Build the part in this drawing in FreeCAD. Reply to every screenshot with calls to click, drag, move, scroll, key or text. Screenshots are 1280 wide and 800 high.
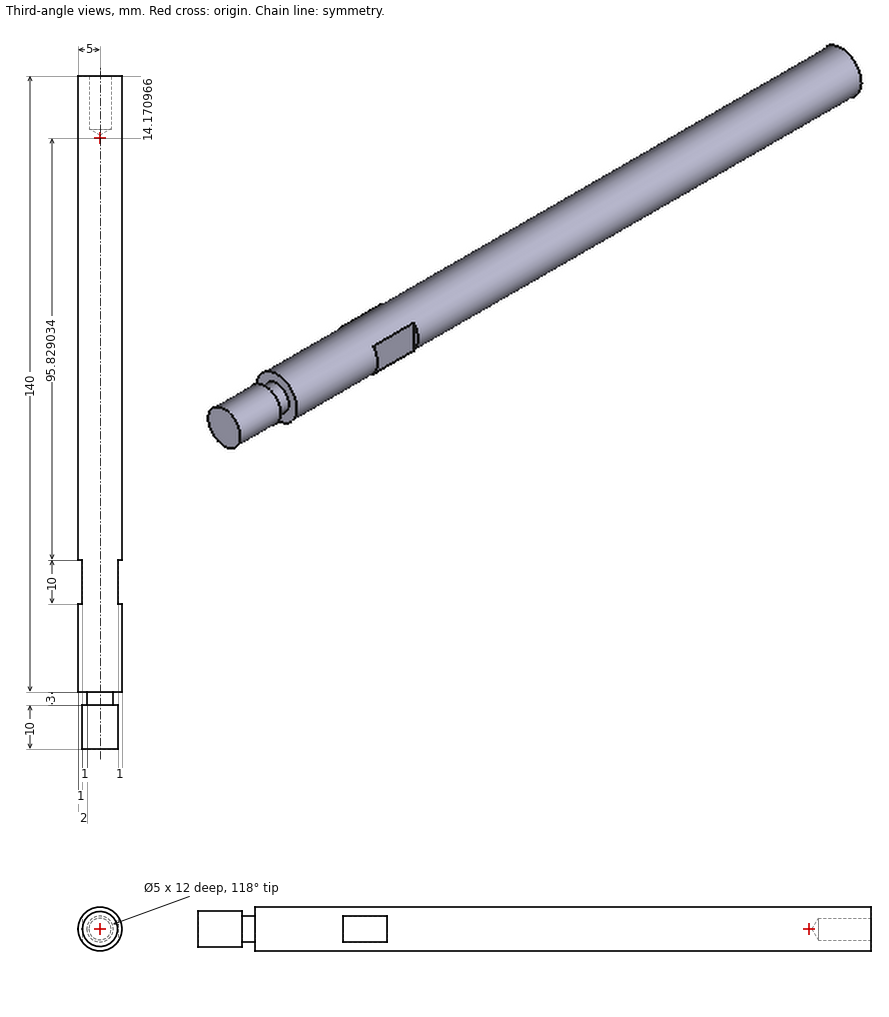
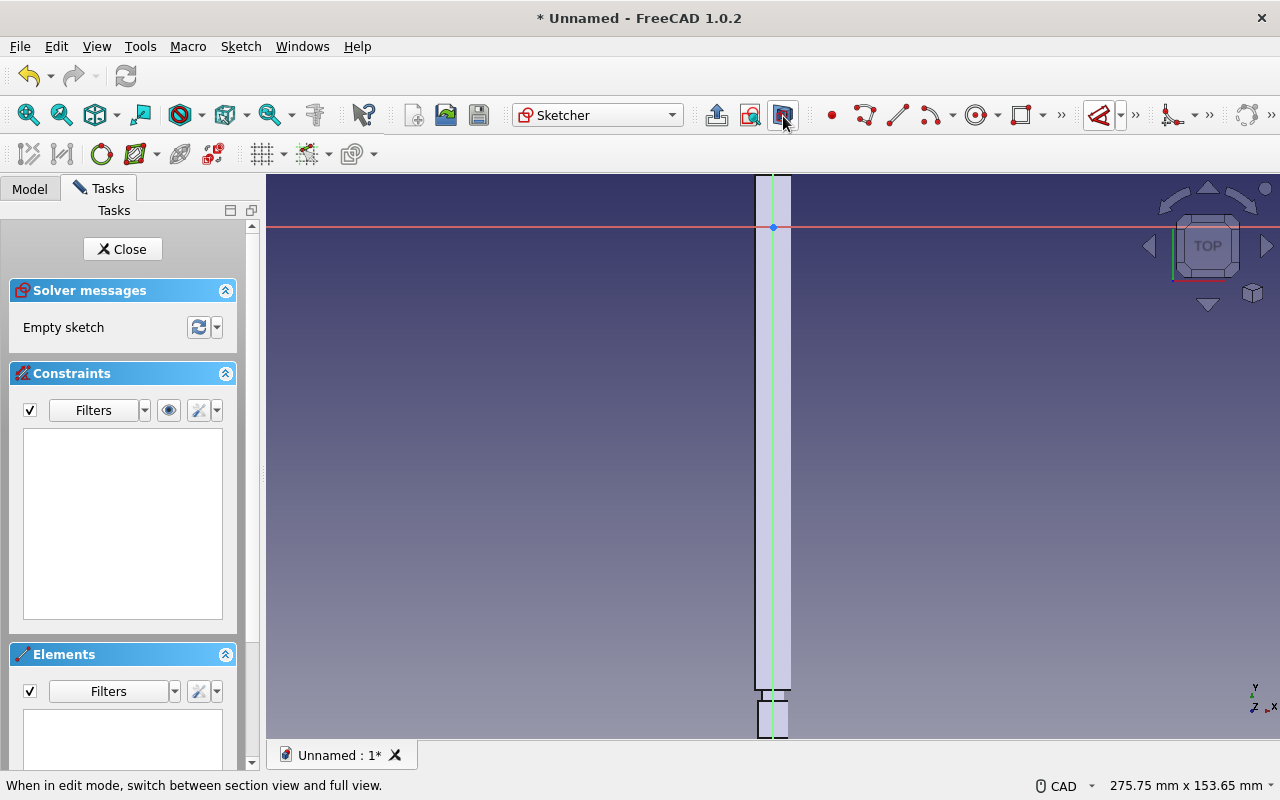
scroll(782, 616, up, 11)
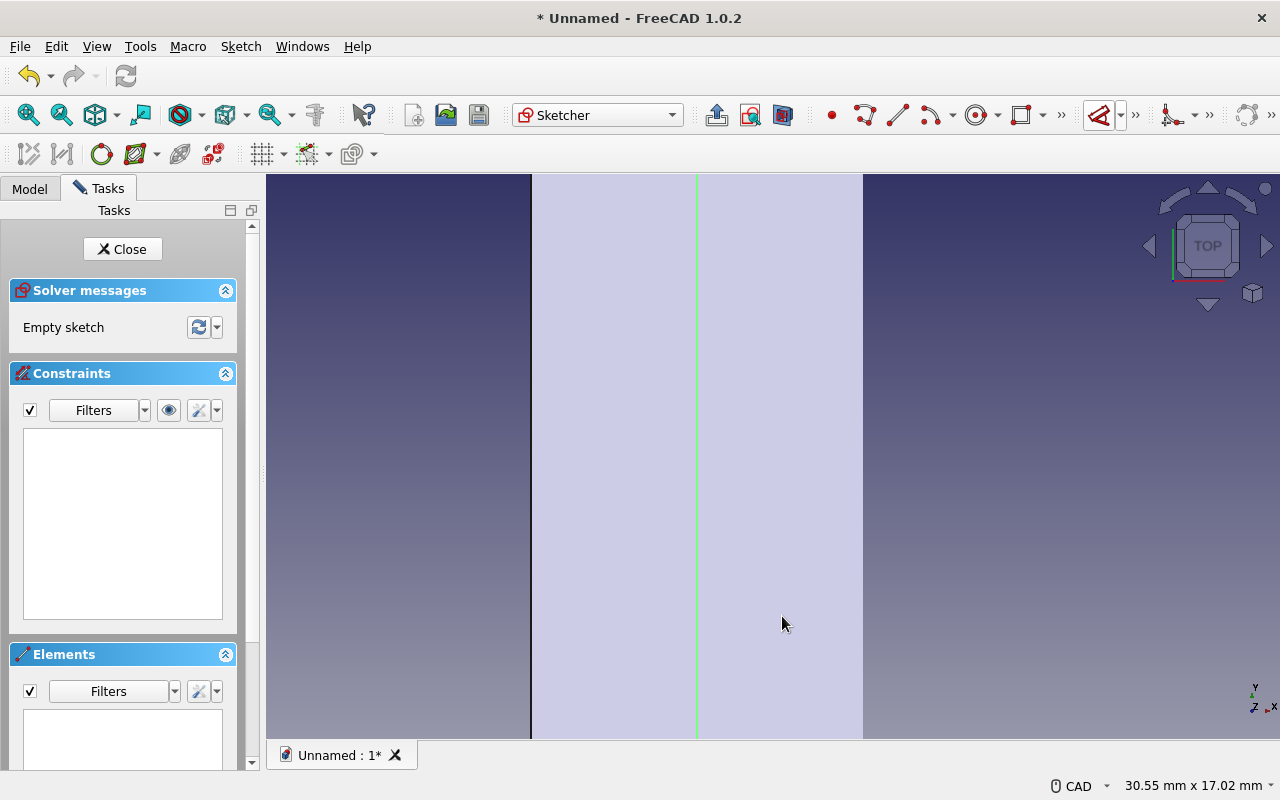
click(1020, 116)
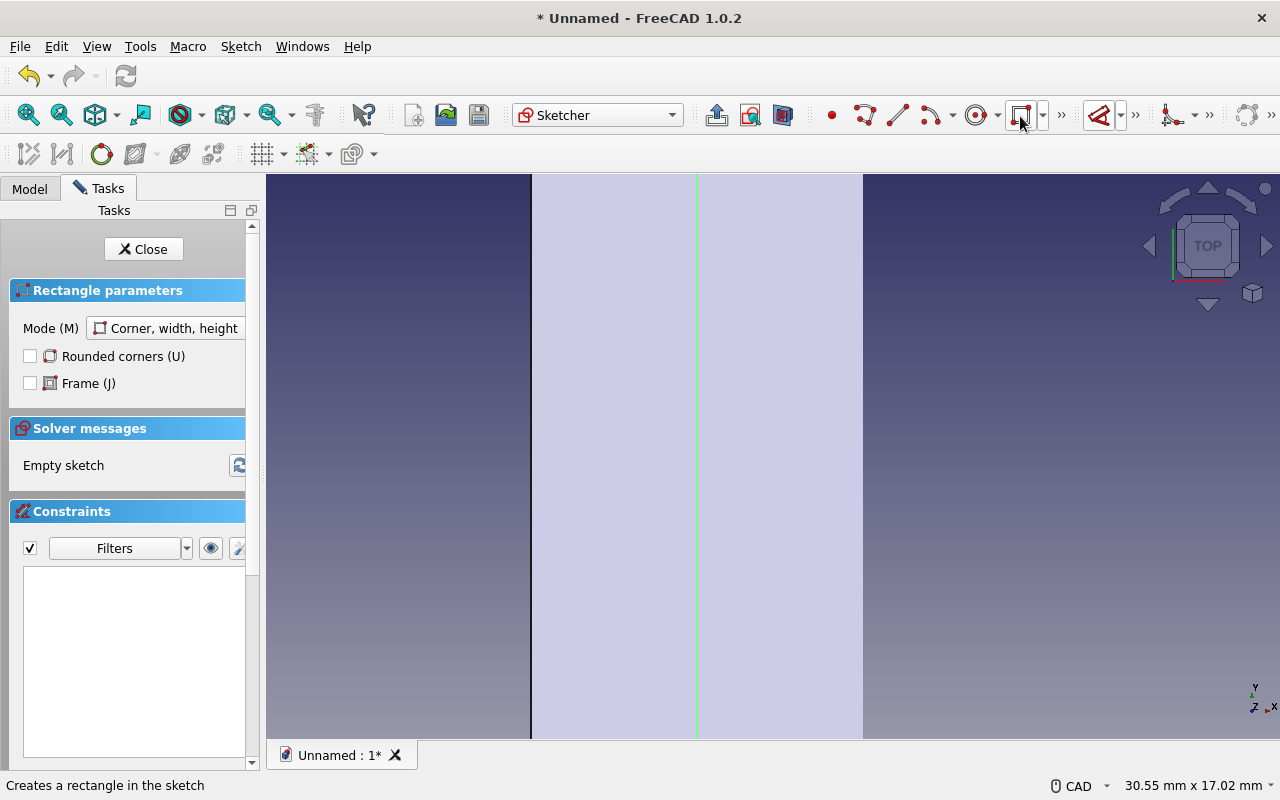
click(531, 282)
move(564, 614)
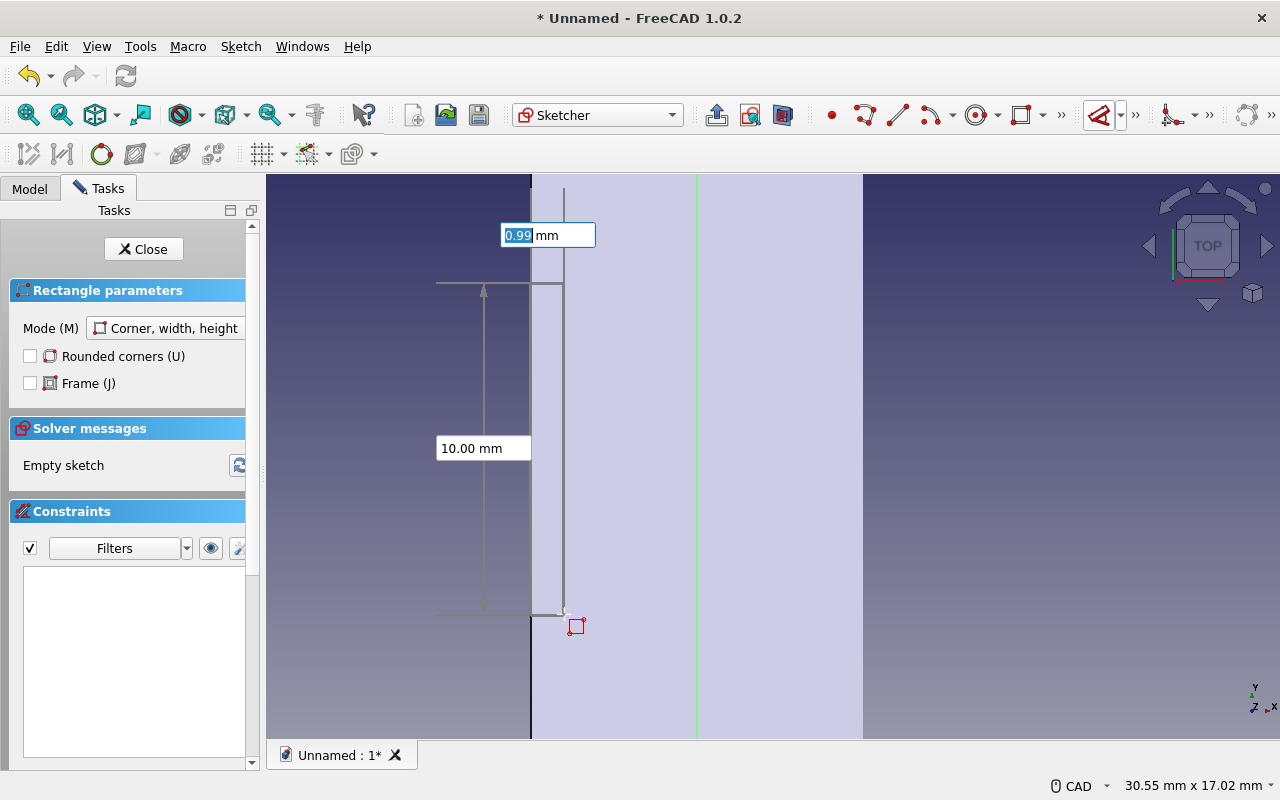
text(1)
key(Tab)
text(10)
key(Return)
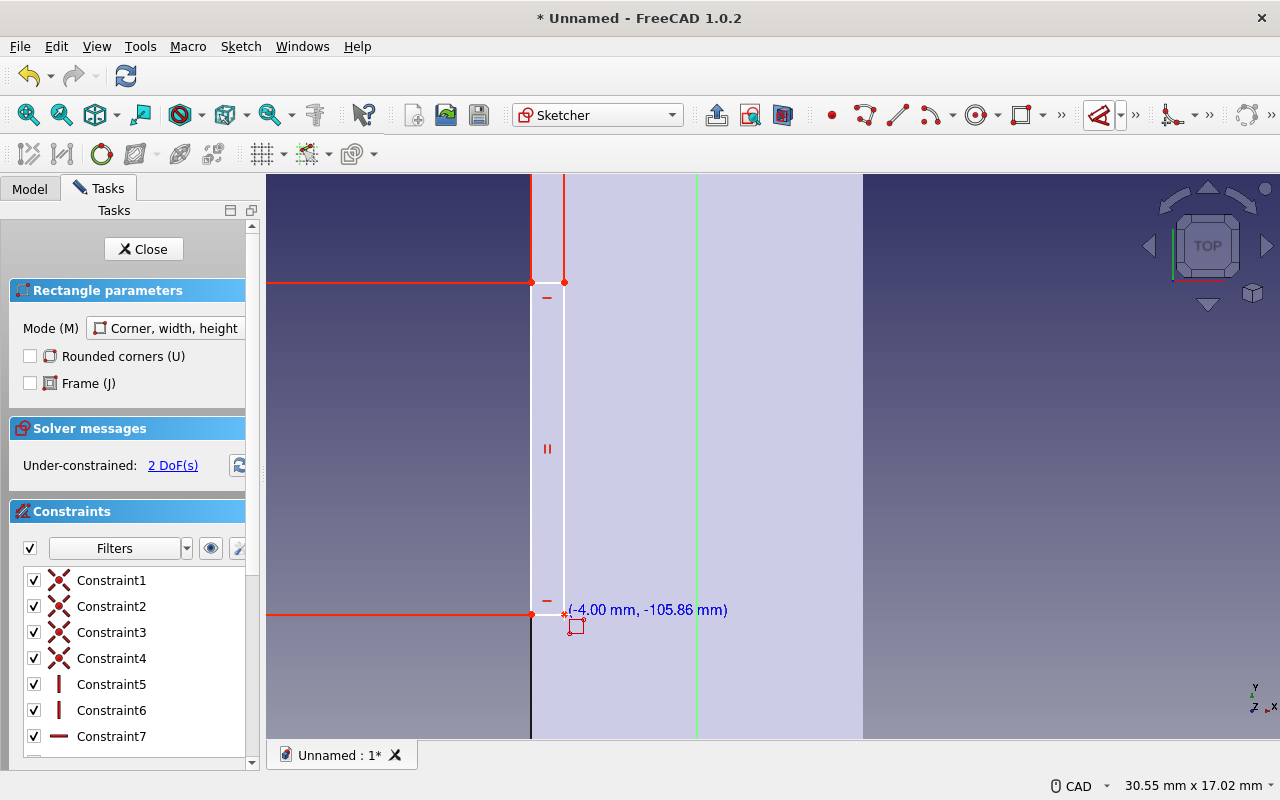
click(829, 282)
move(863, 614)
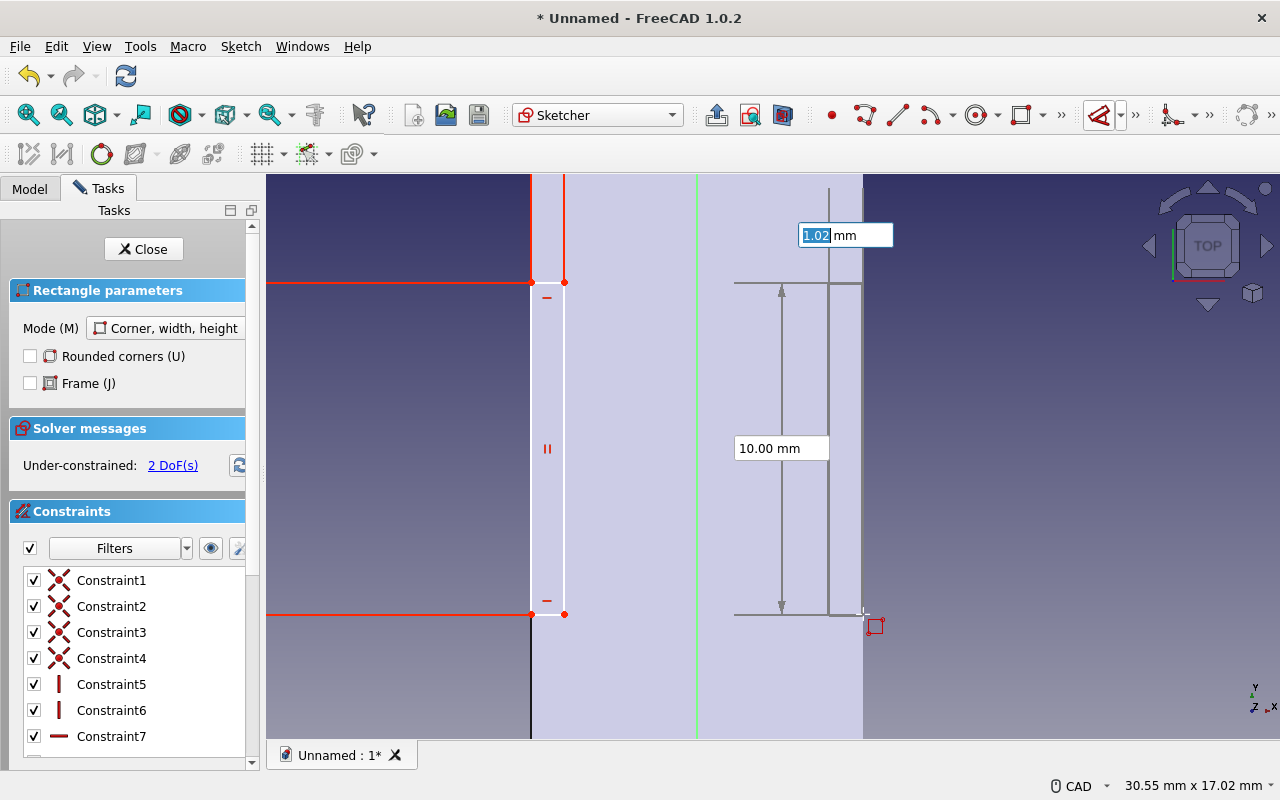
text(1)
key(Tab)
text(10)
key(Return)
key(Escape)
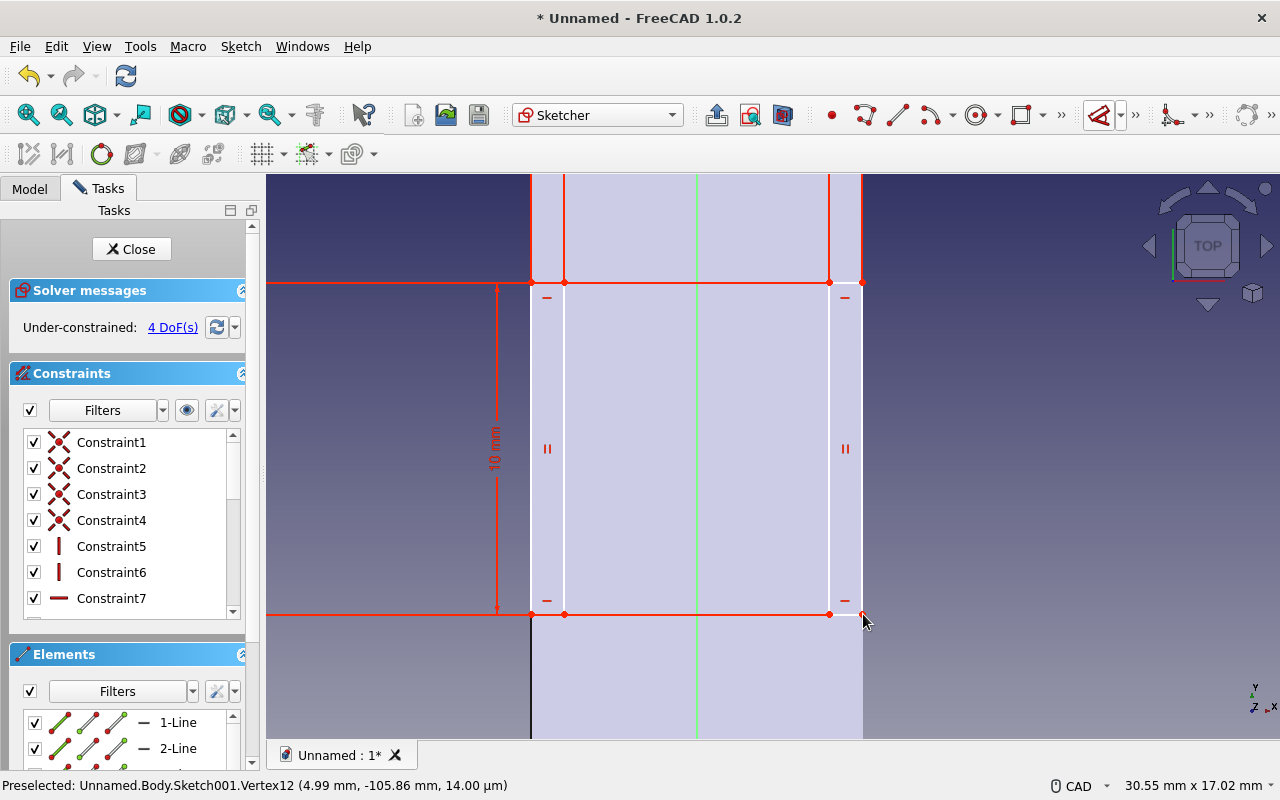
click(564, 283)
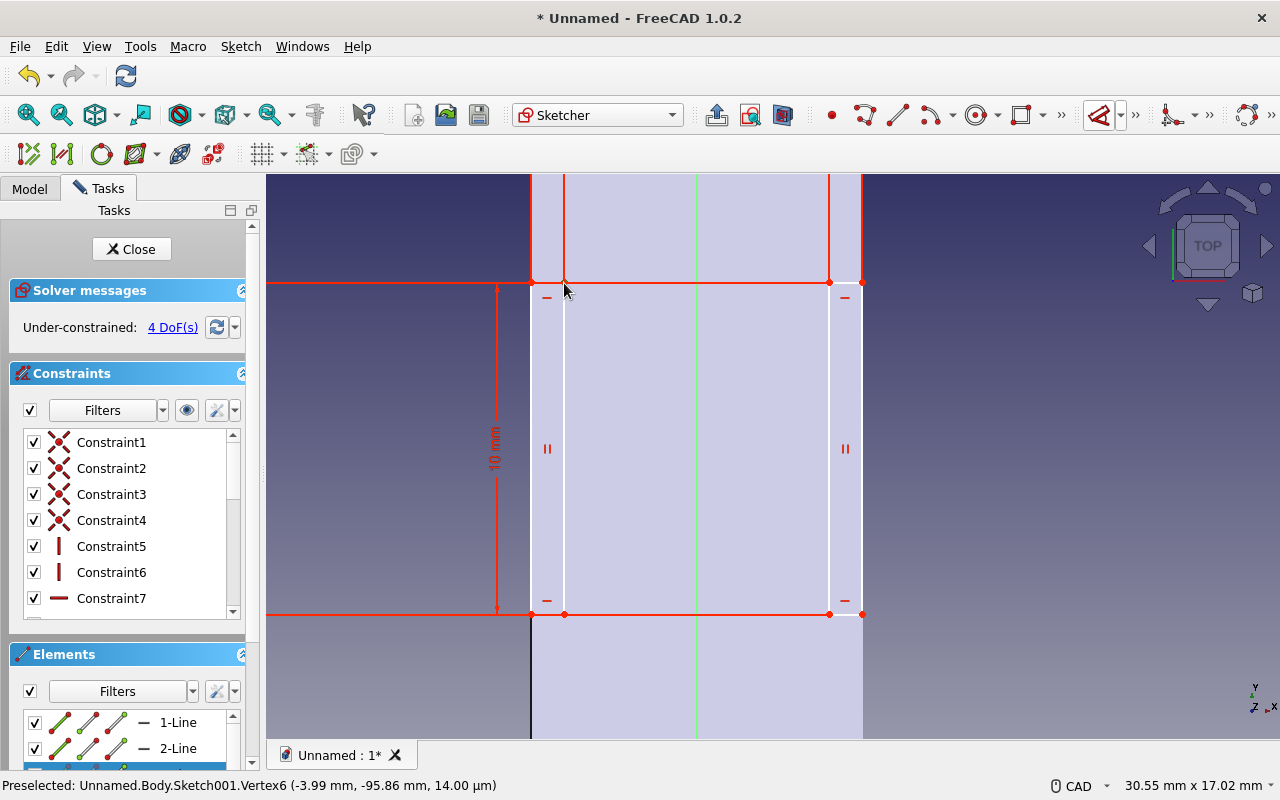
click(829, 283)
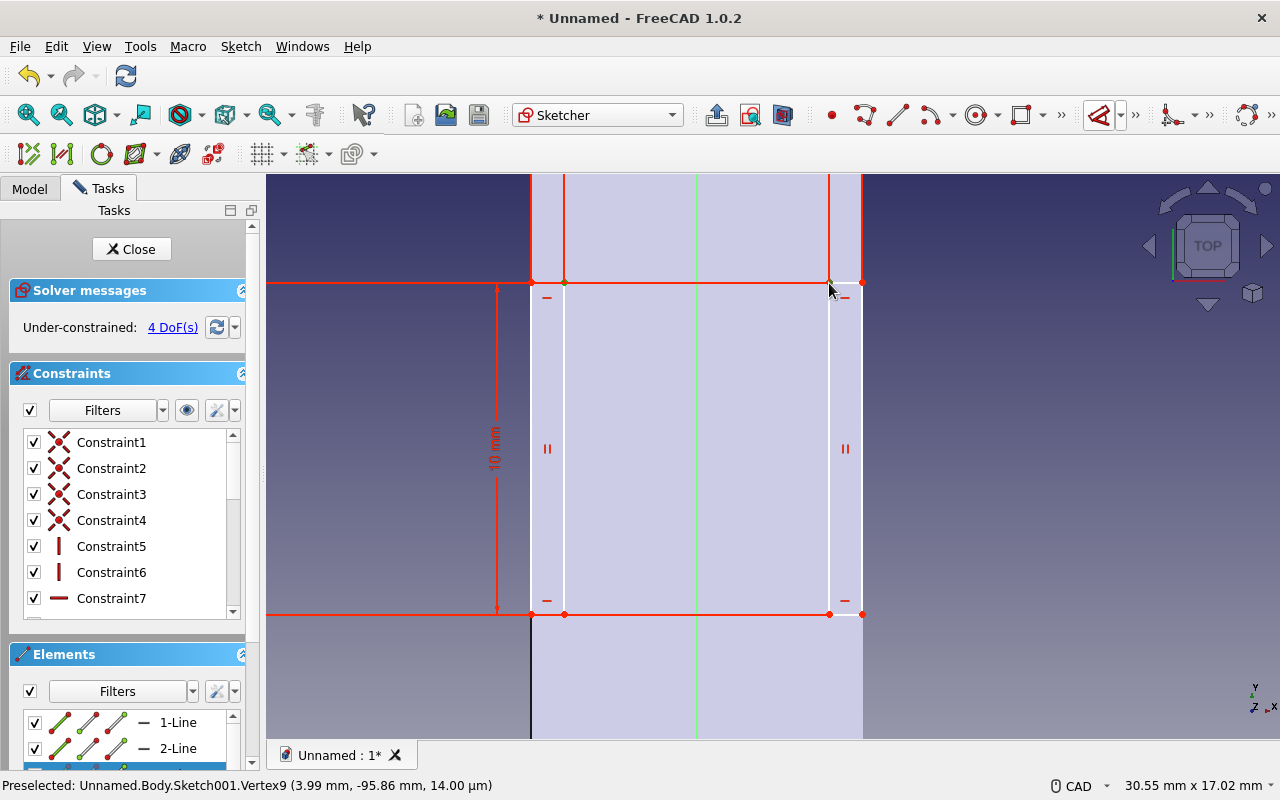
click(697, 675)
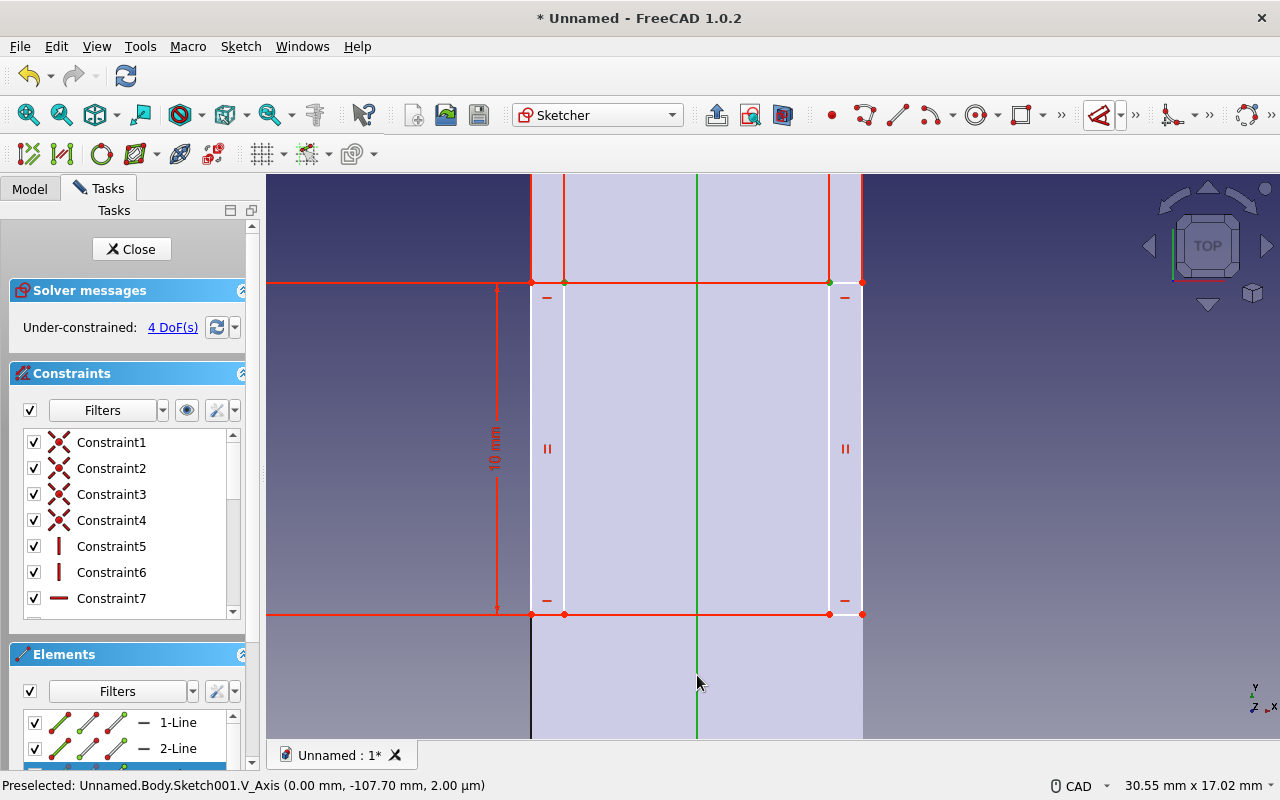
key(s)